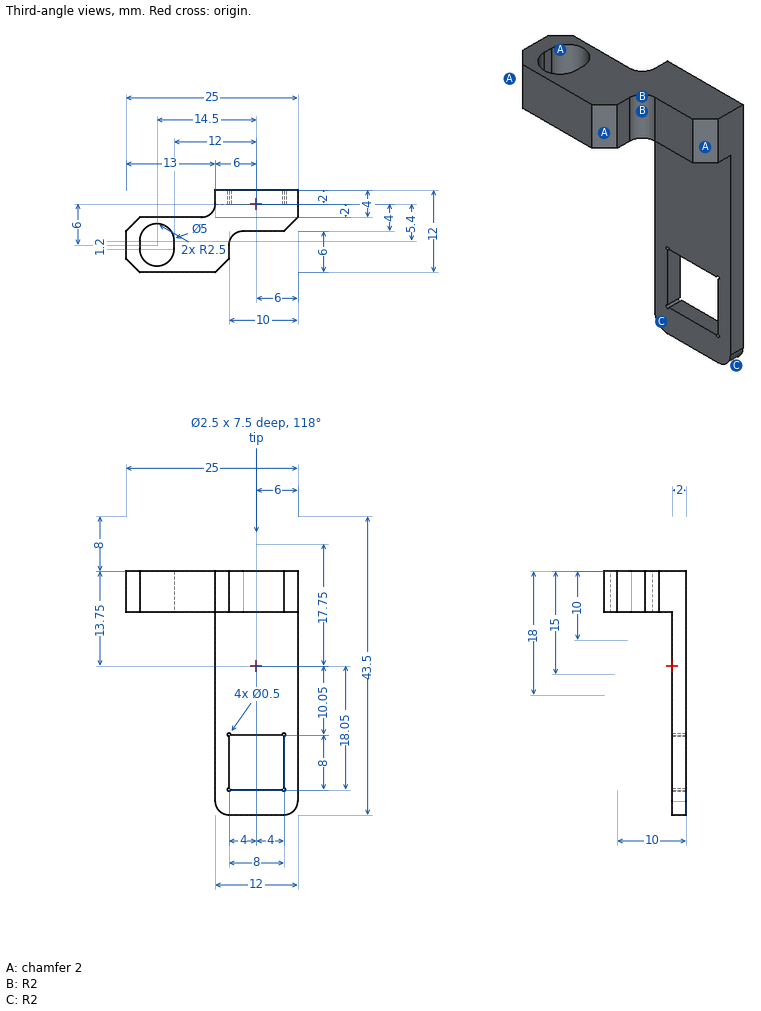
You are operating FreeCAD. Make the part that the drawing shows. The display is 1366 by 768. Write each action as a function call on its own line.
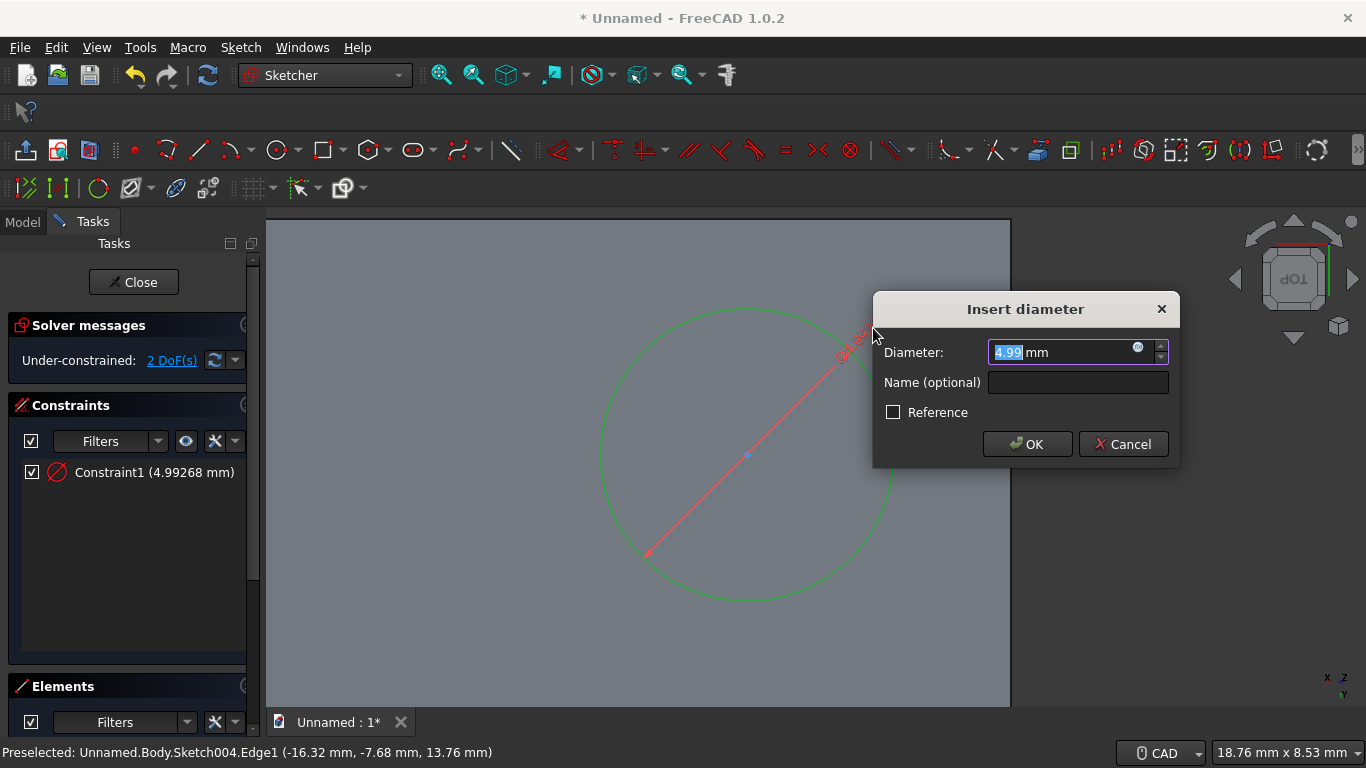
text(5)
key(Return)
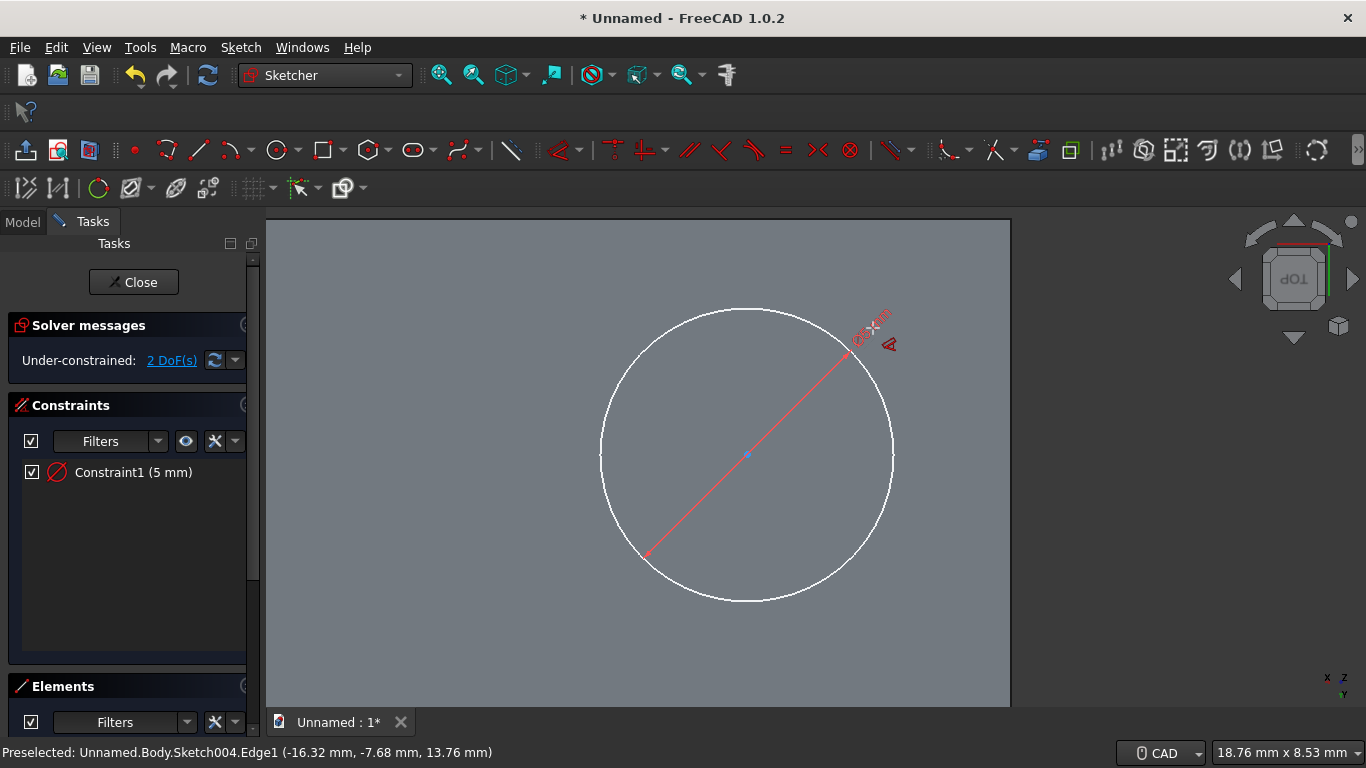
click(747, 455)
click(781, 567)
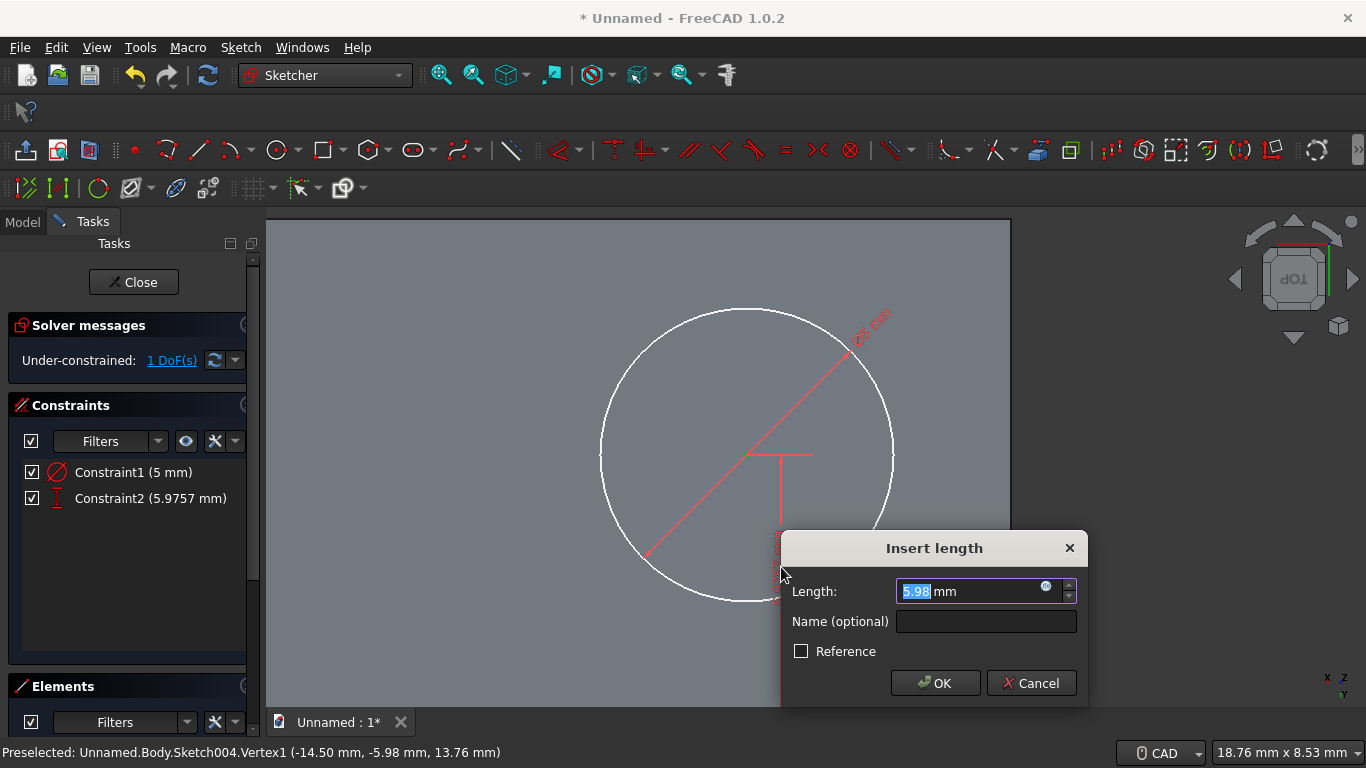
text(6)
key(Return)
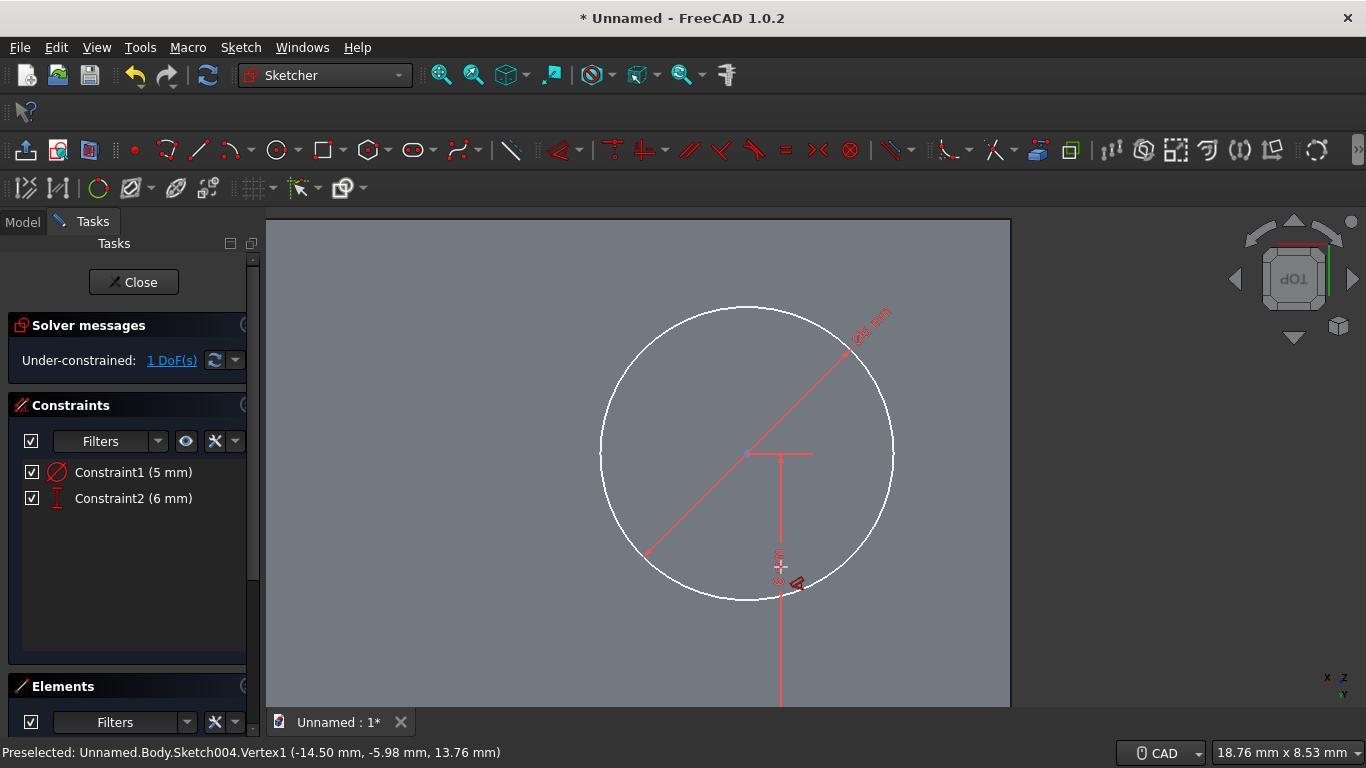
click(747, 454)
click(520, 420)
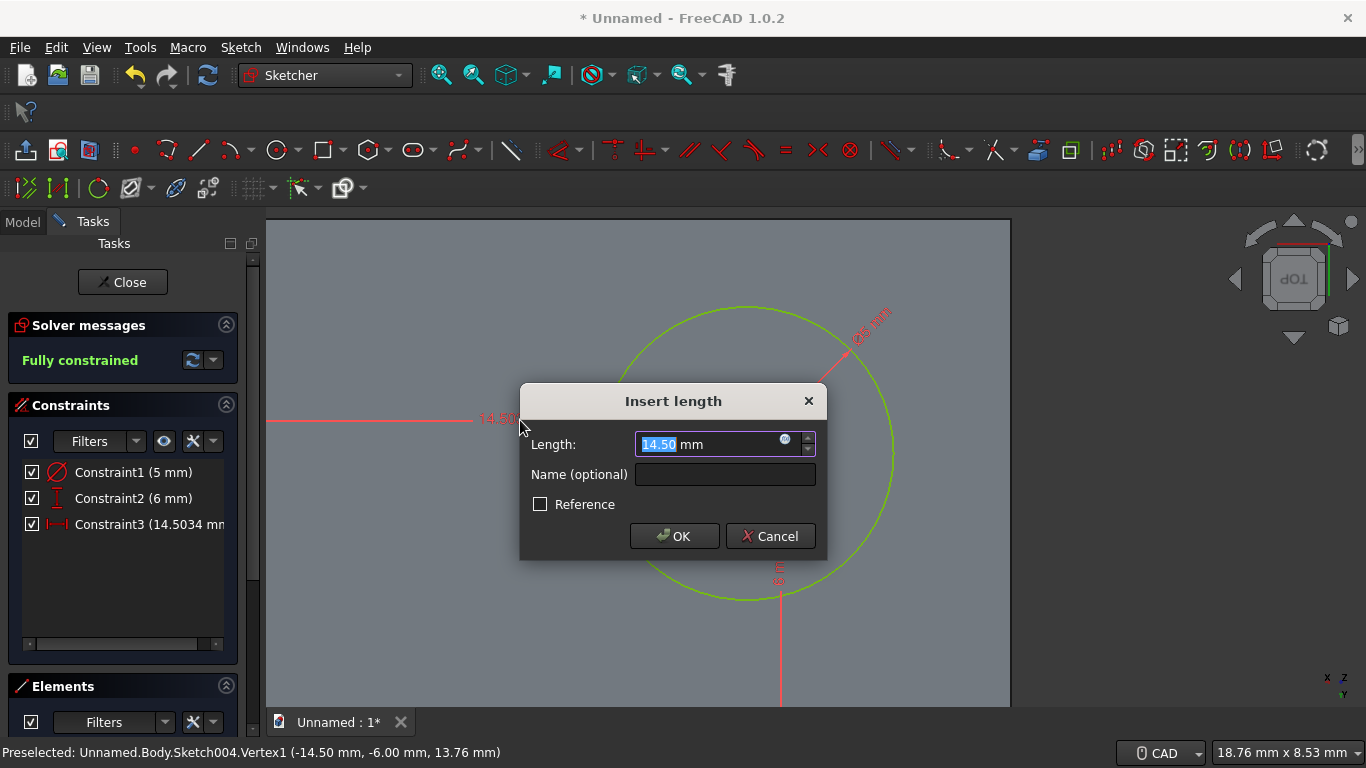
text(14.5)
key(Return)
key(Escape)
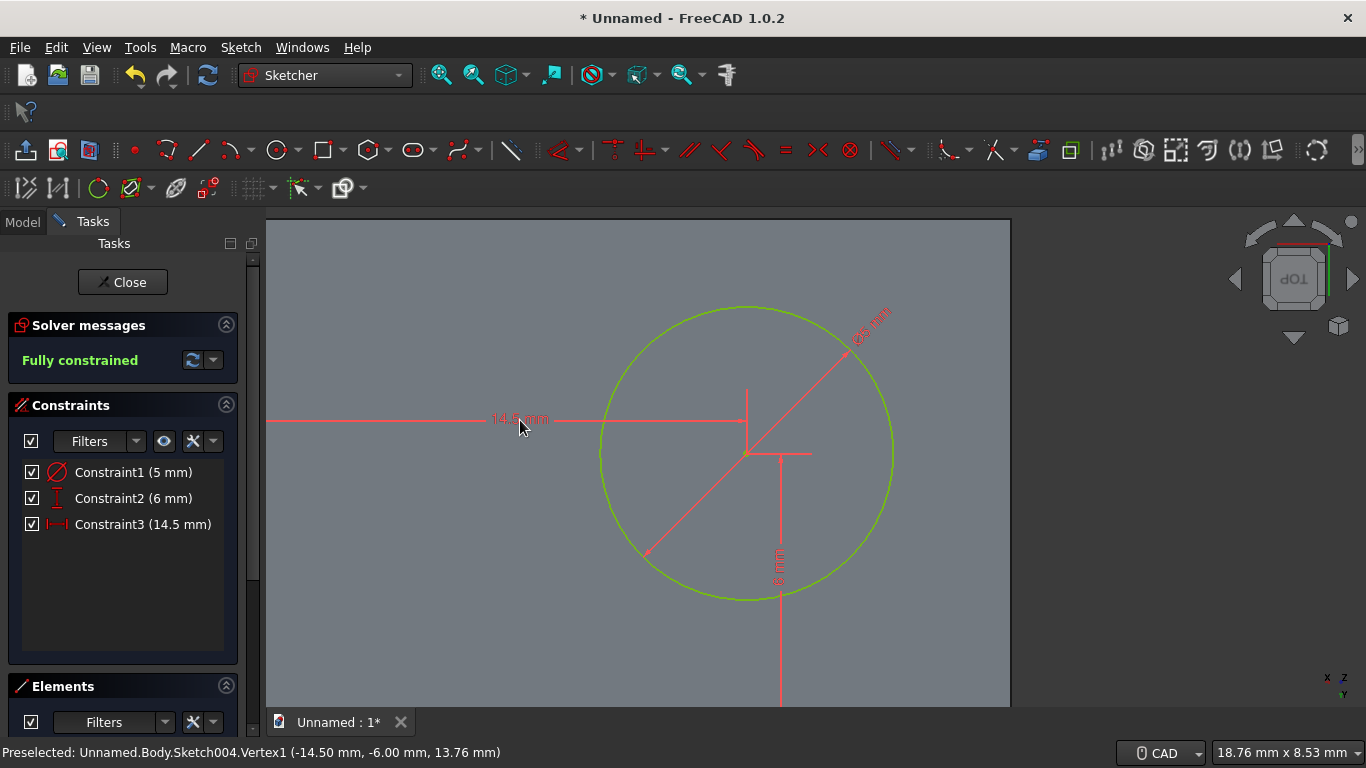
click(123, 282)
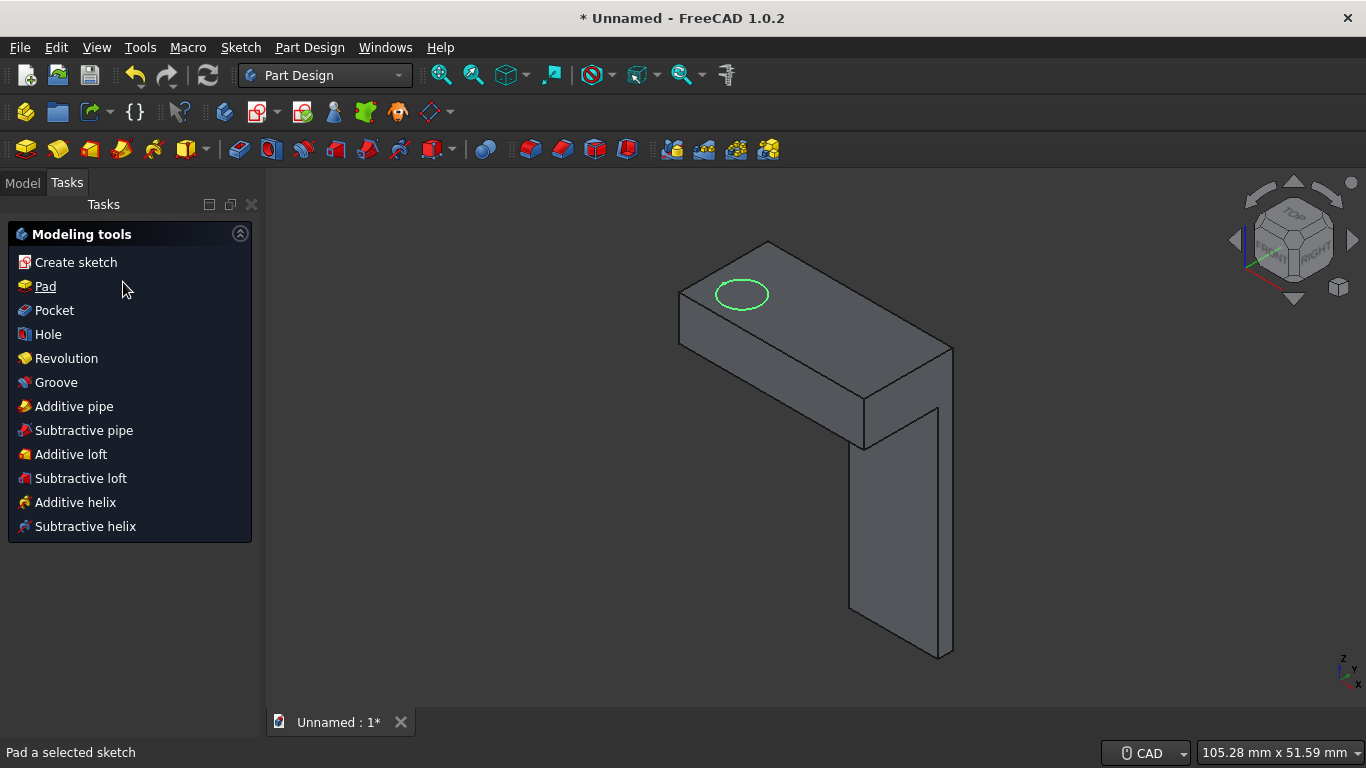
click(240, 150)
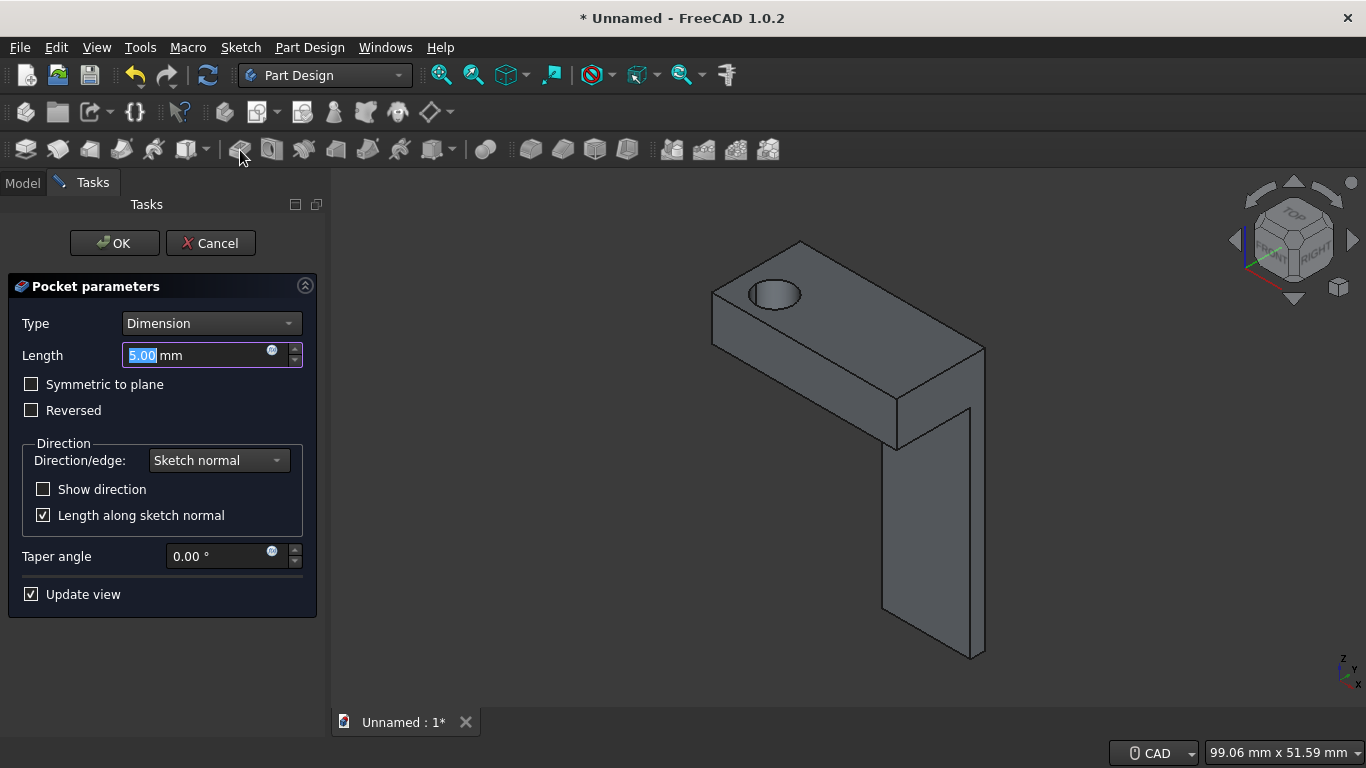
text(15)
key(Tab)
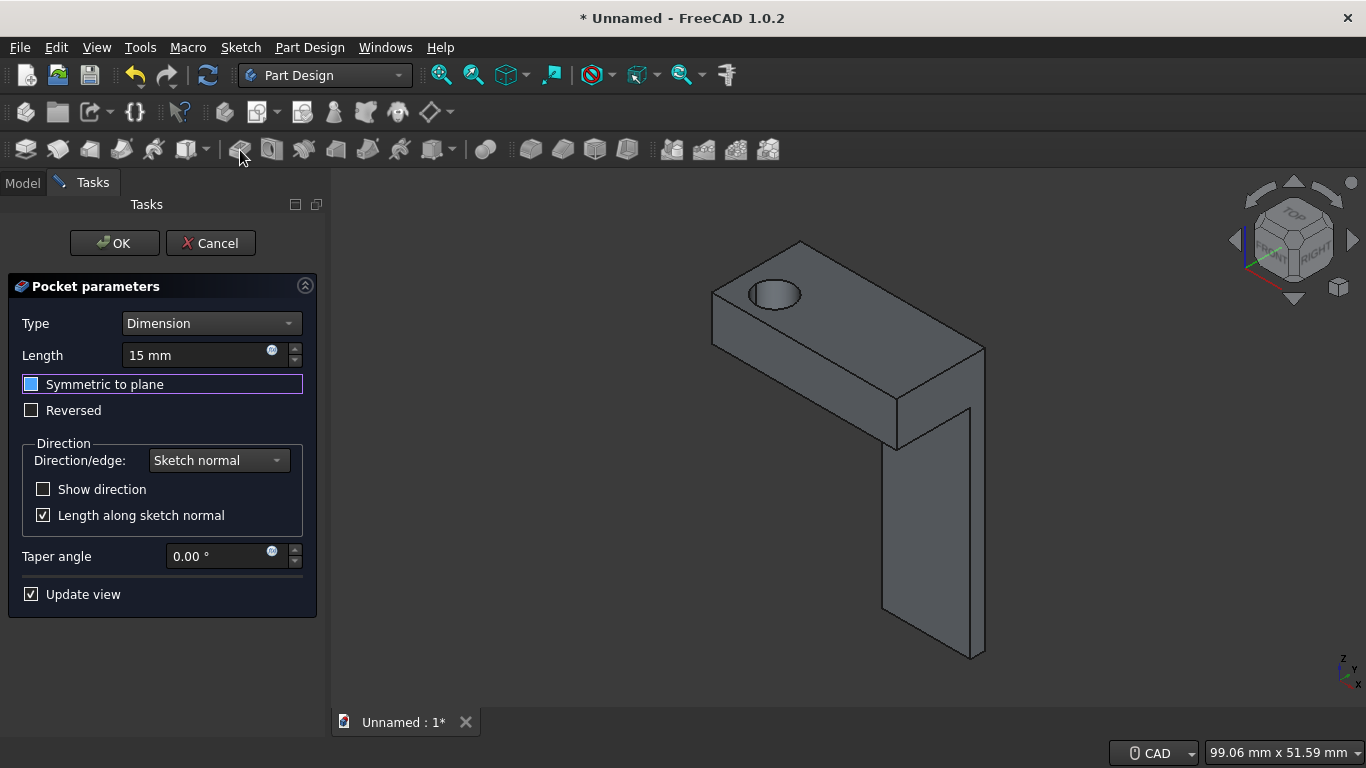
click(115, 243)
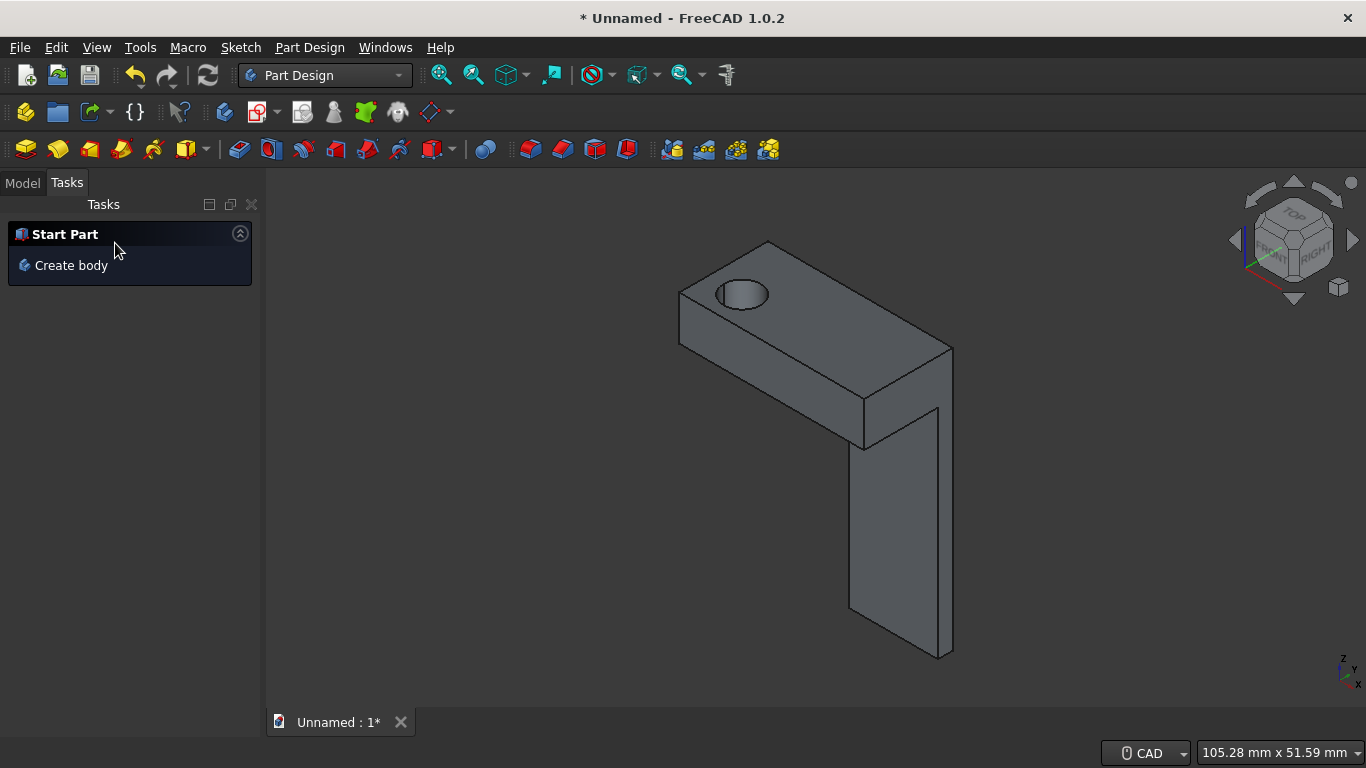
click(842, 334)